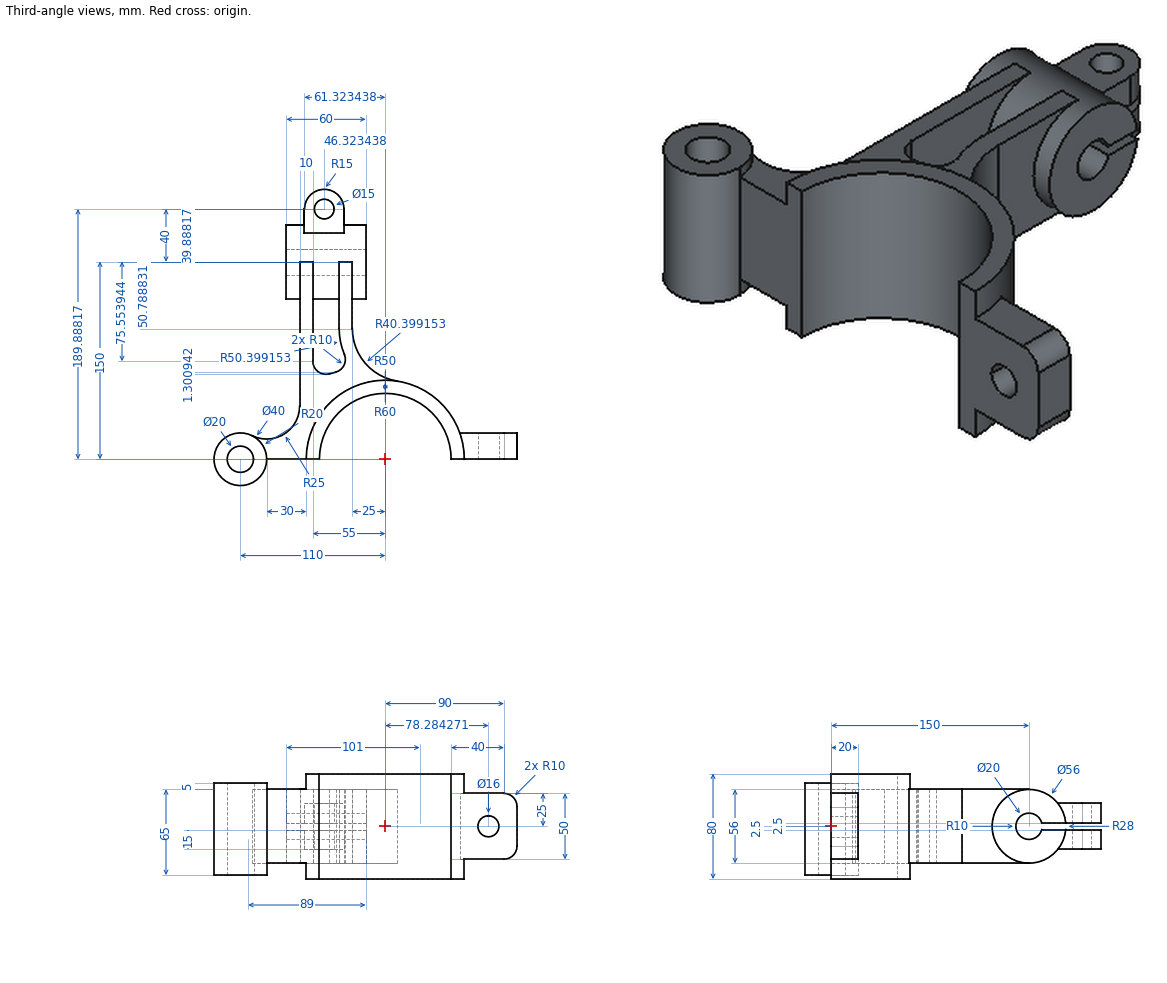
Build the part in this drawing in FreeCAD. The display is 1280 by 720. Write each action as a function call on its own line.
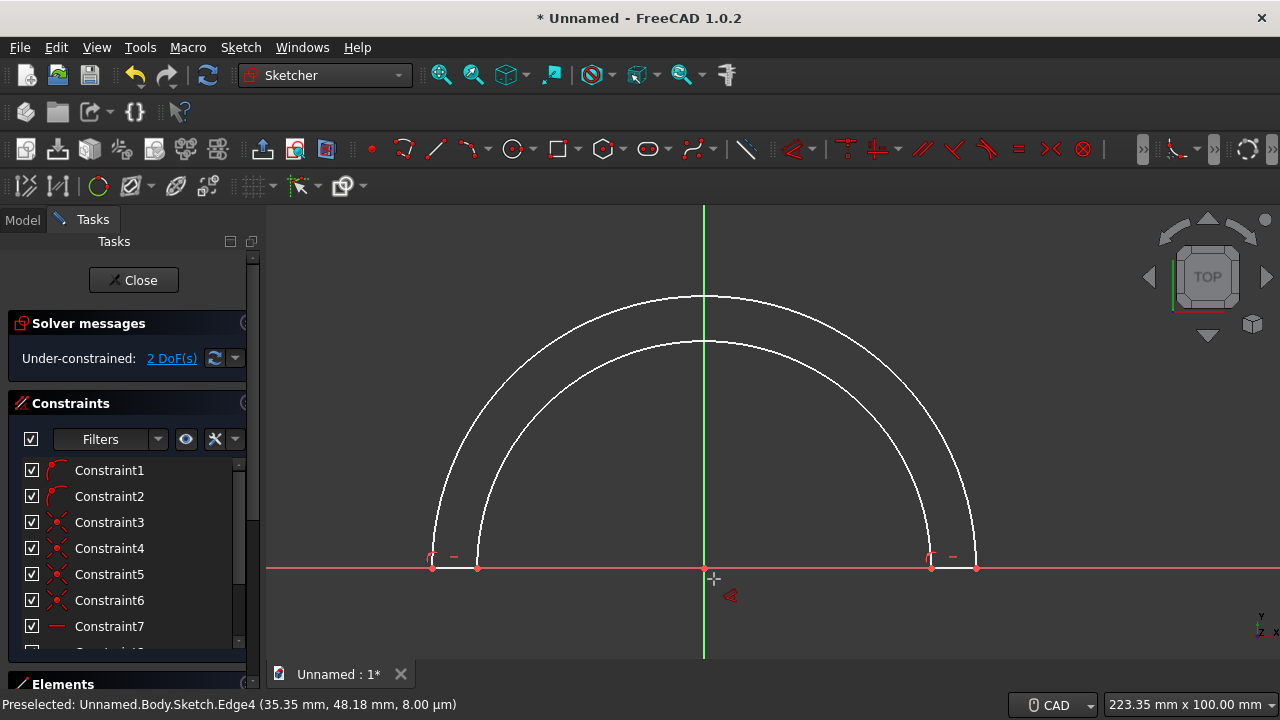
click(837, 384)
click(963, 582)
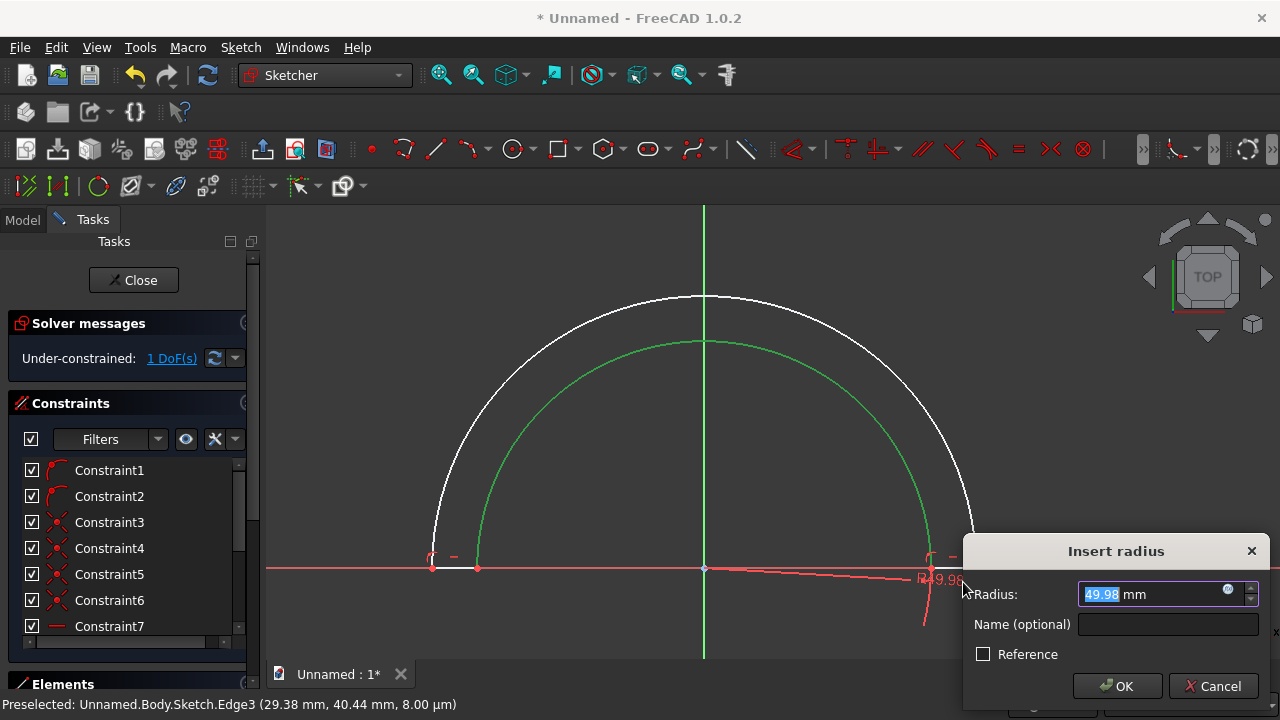
text(50)
key(Return)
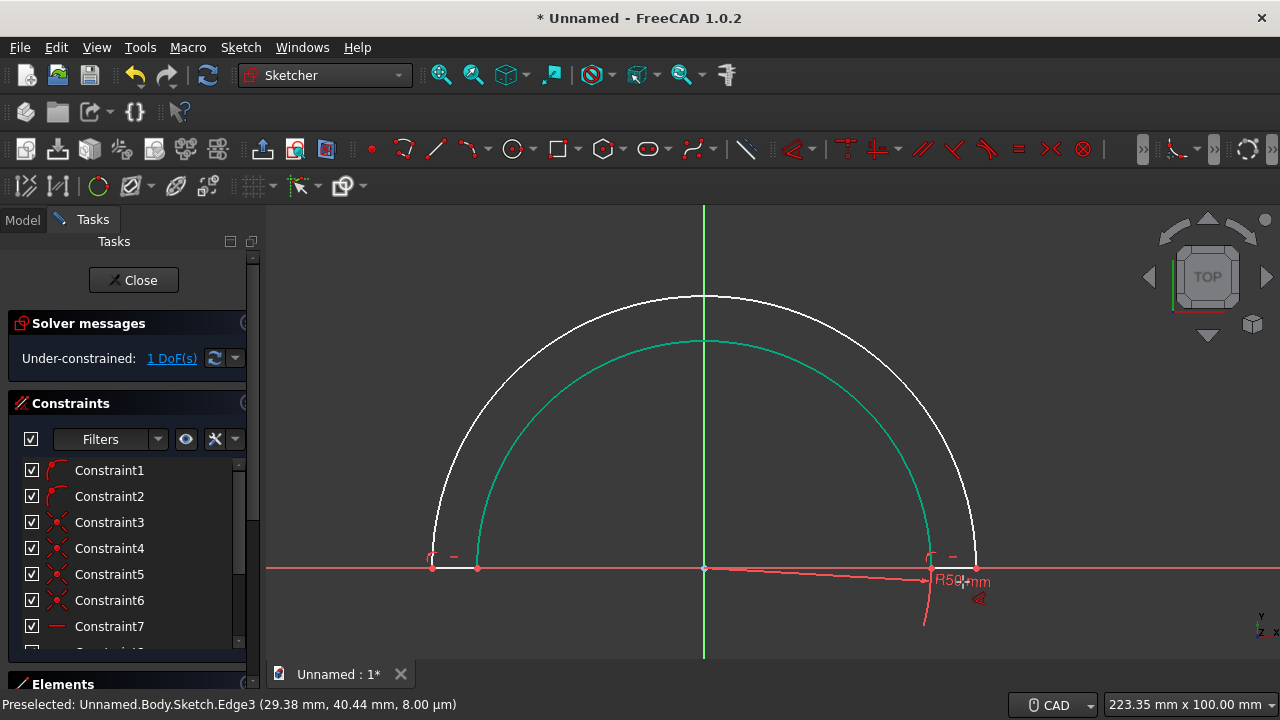
click(864, 348)
click(883, 322)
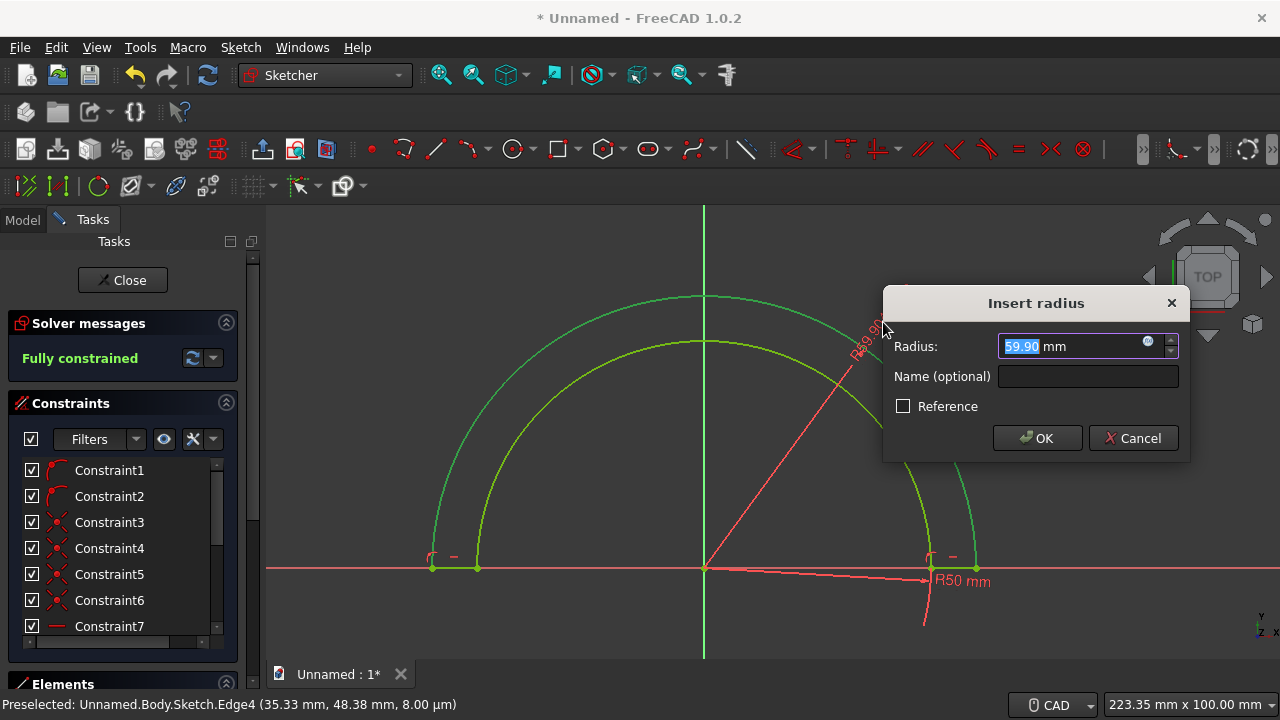
text(60)
key(Return)
key(Escape)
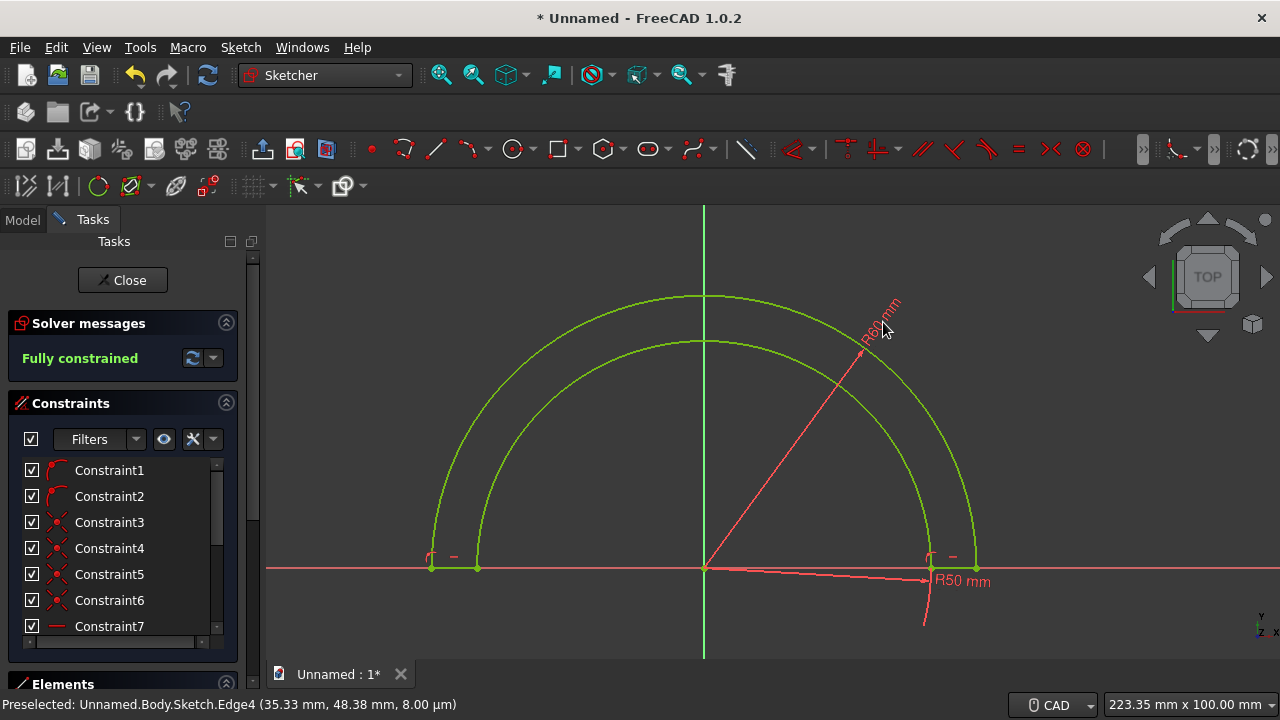
click(123, 280)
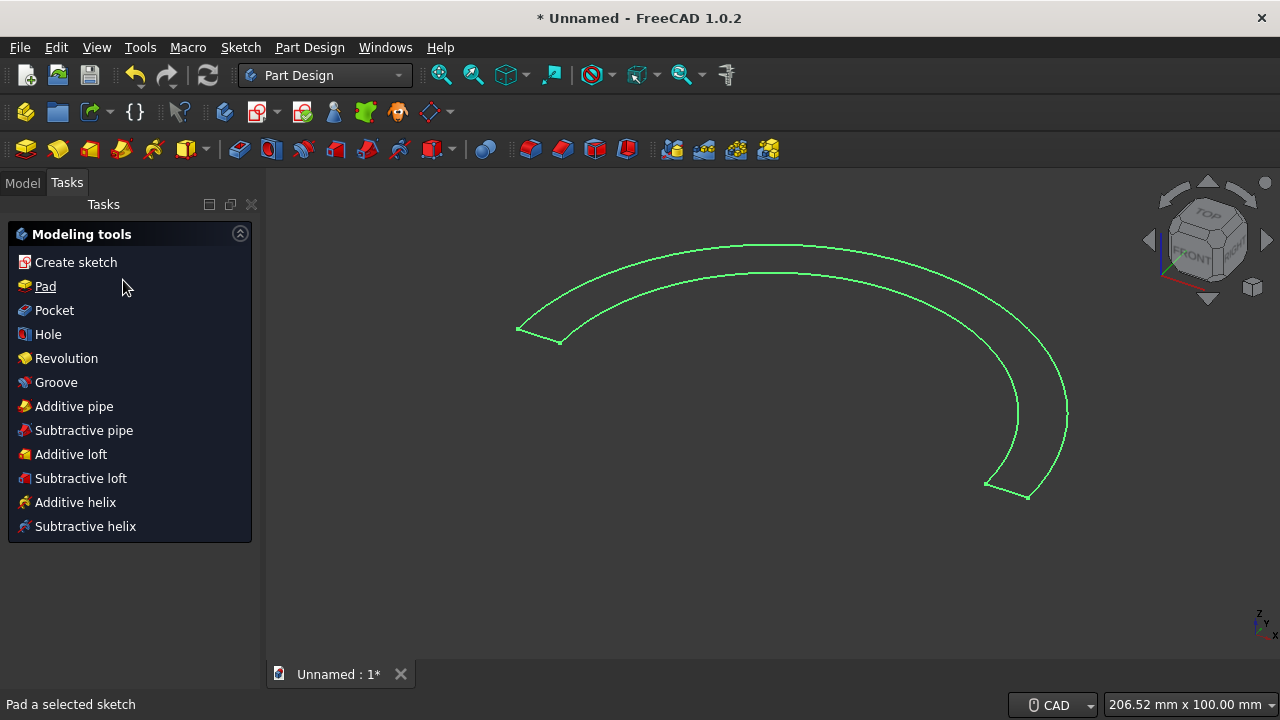
click(26, 150)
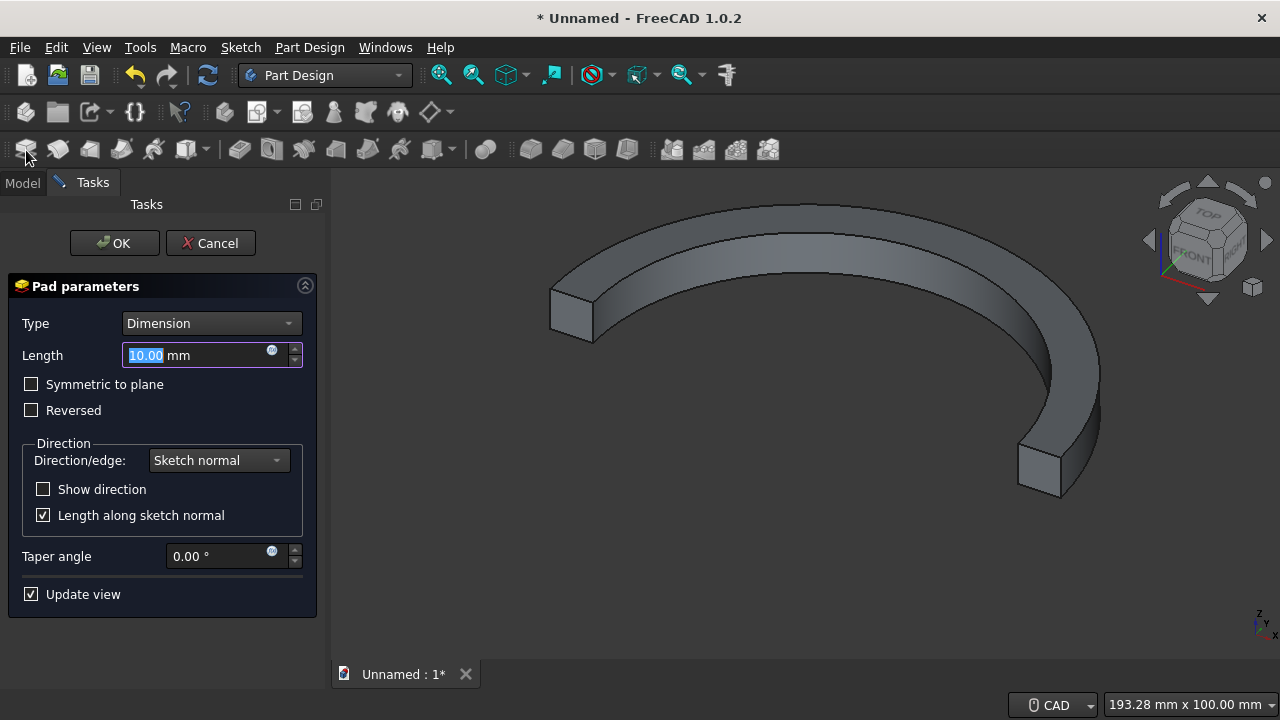
text(80)
key(Tab)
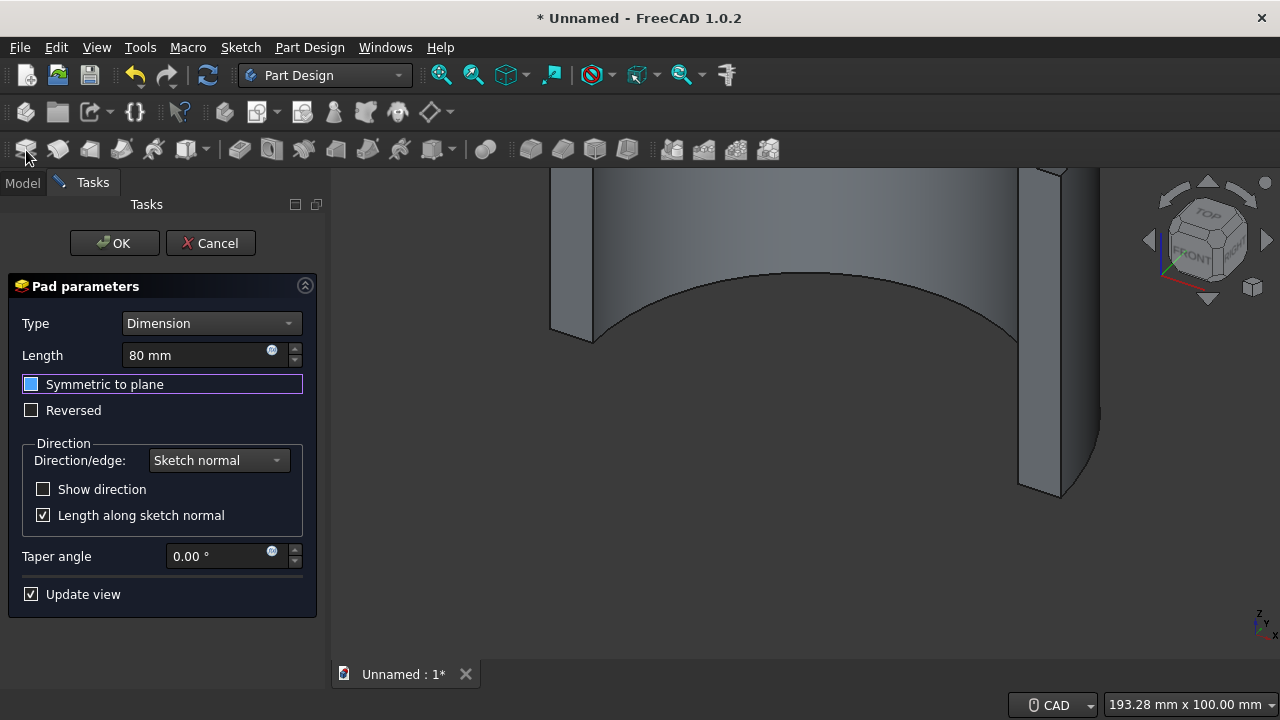
click(30, 384)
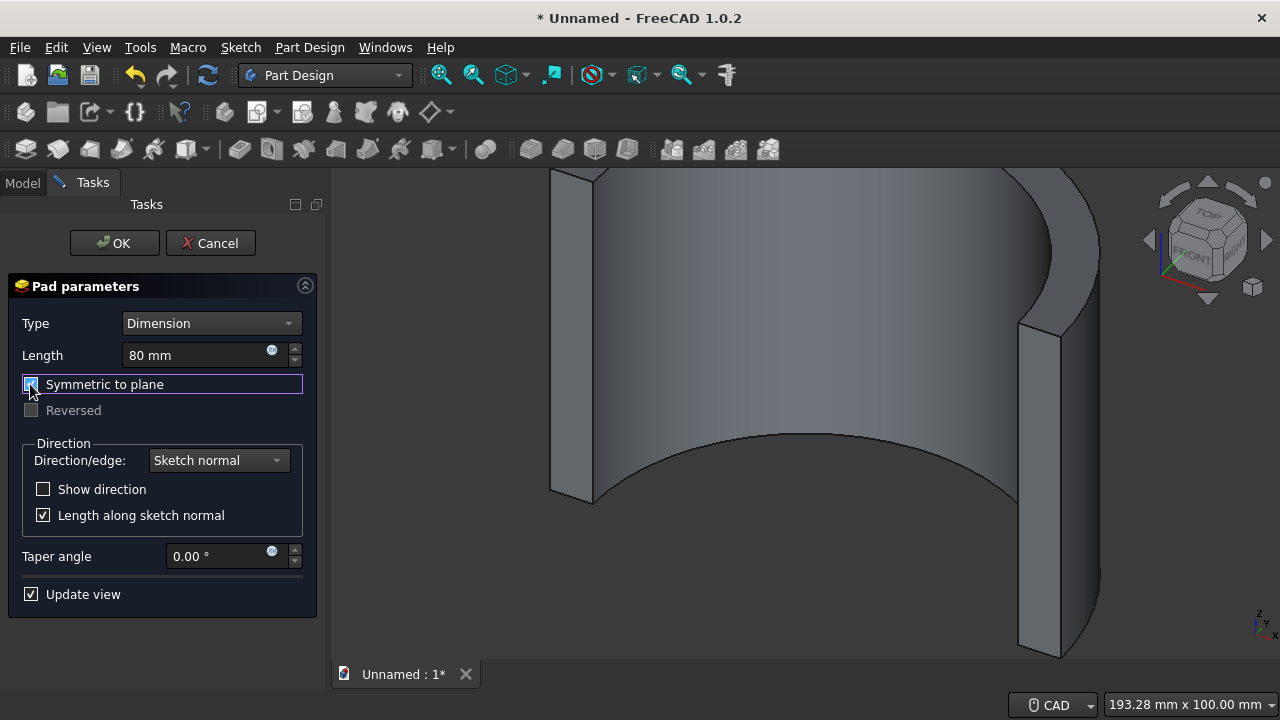
click(115, 243)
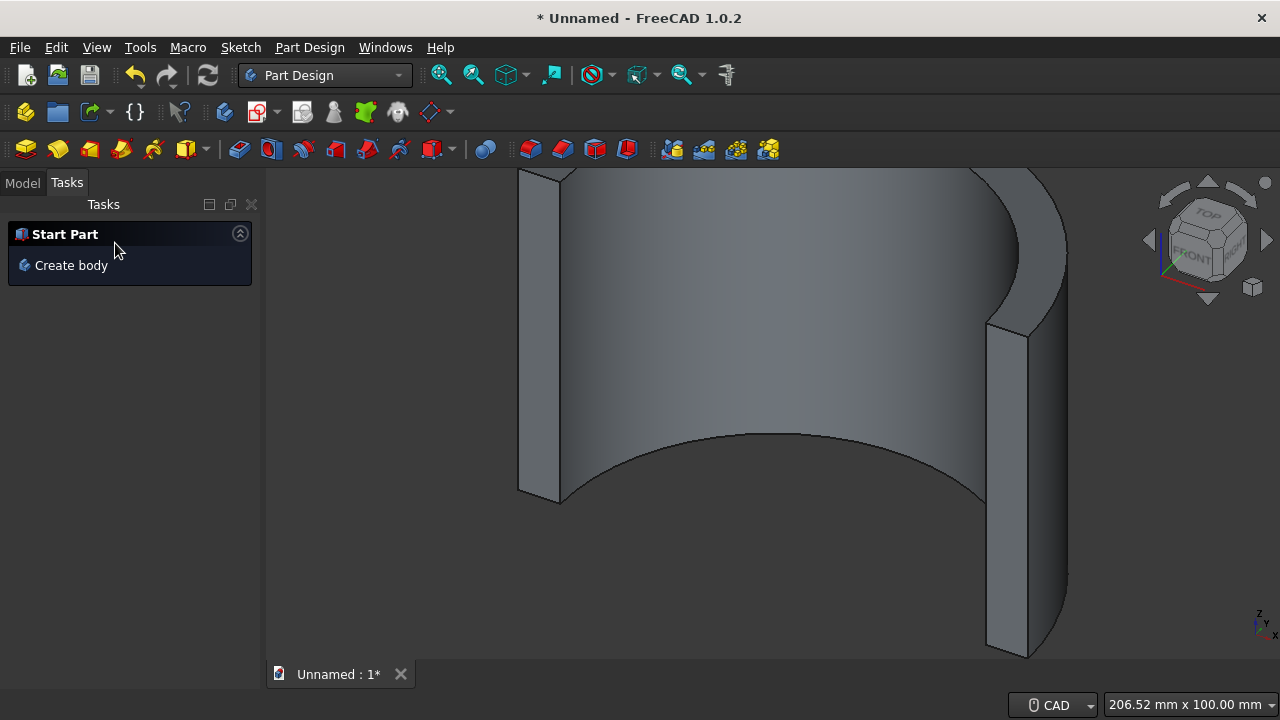
click(442, 76)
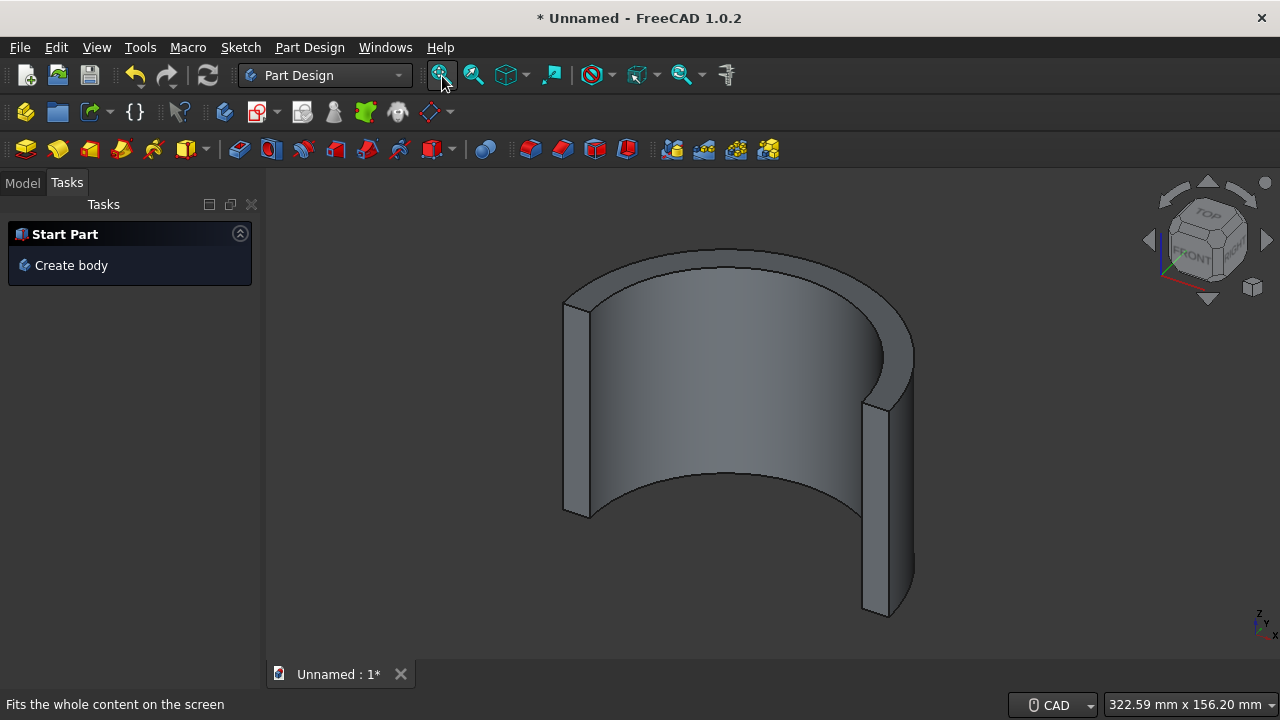
click(226, 112)